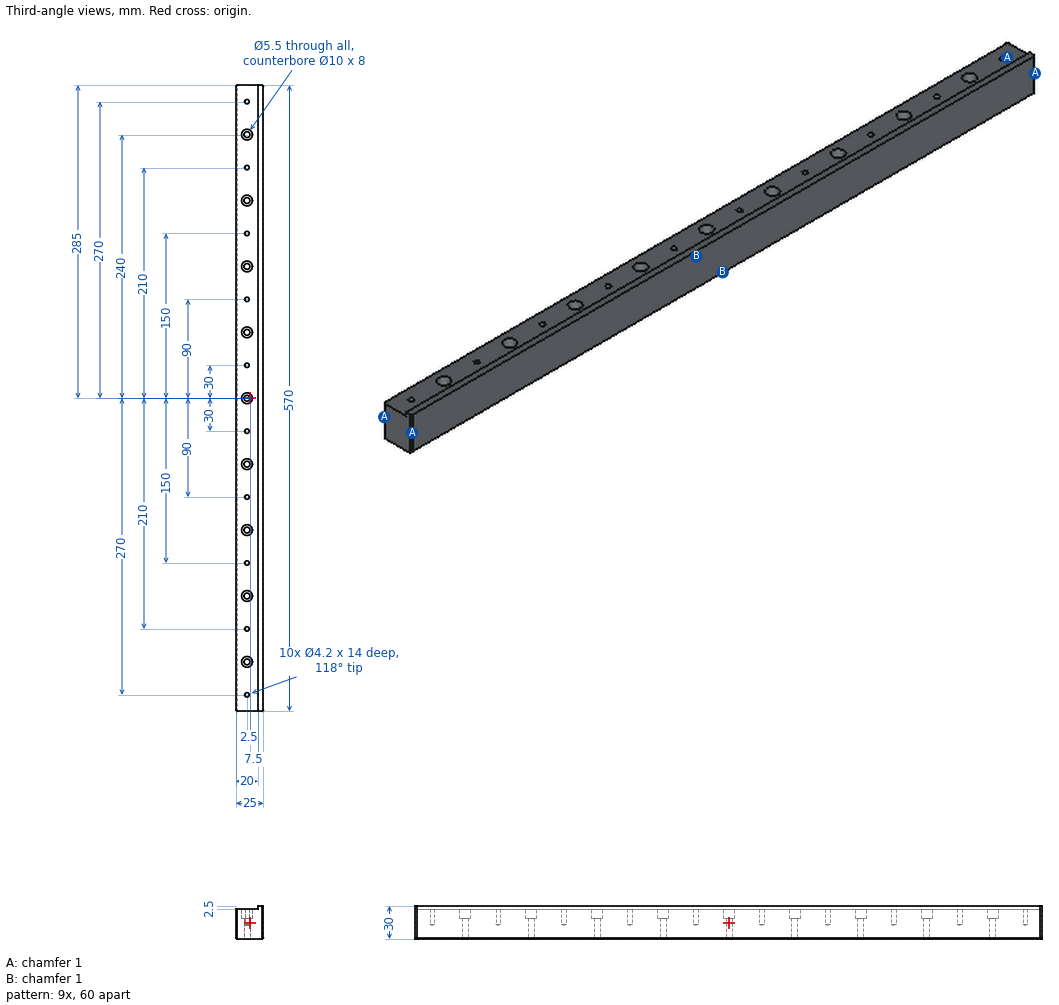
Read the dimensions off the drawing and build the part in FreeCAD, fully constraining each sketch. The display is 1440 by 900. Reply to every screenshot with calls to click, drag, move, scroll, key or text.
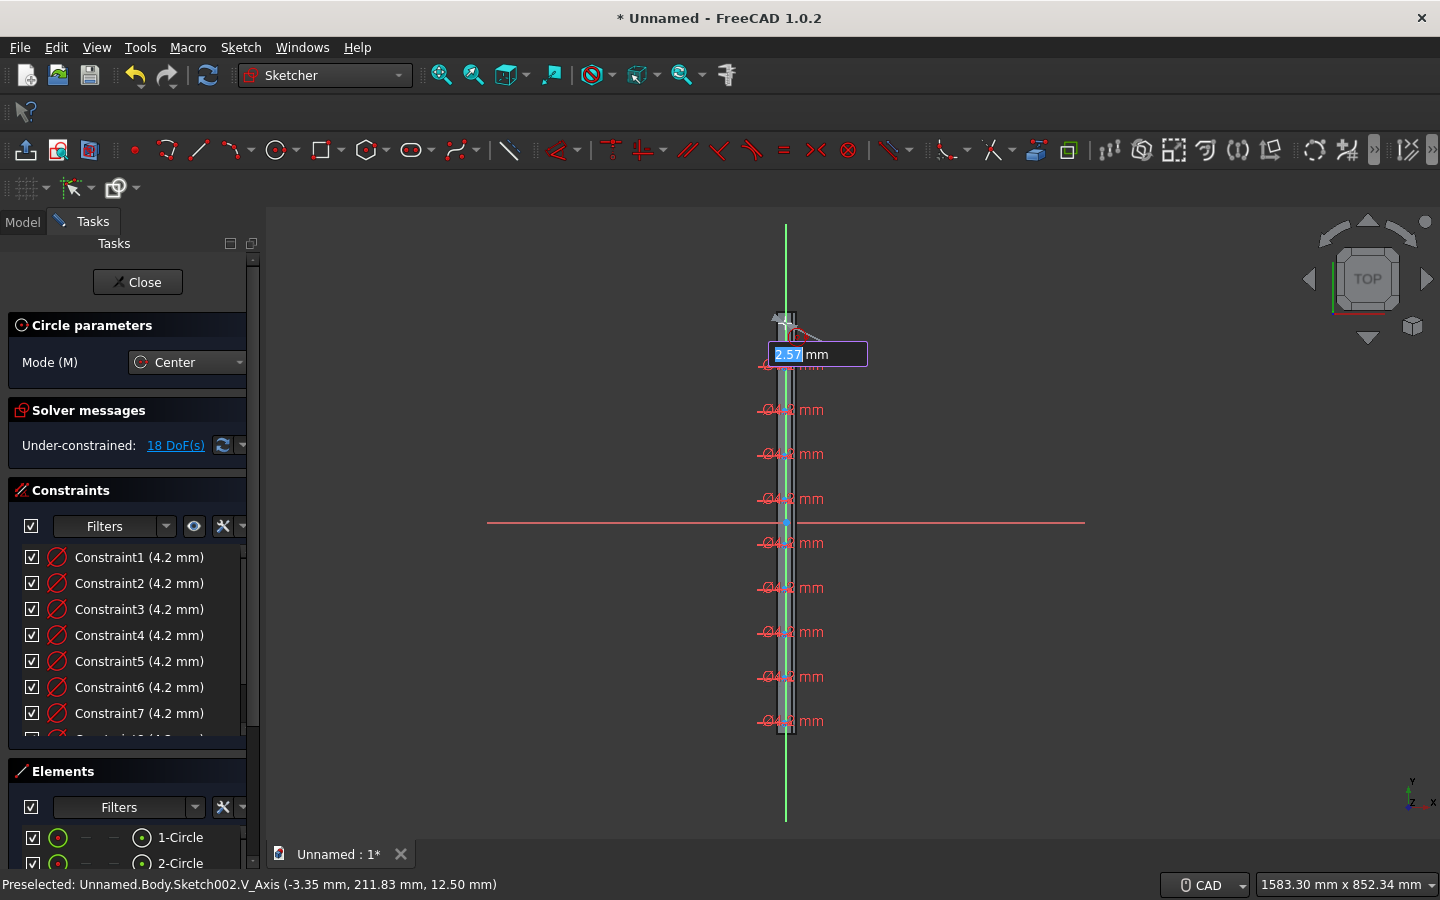
scroll(783, 322, up, 9)
move(783, 319)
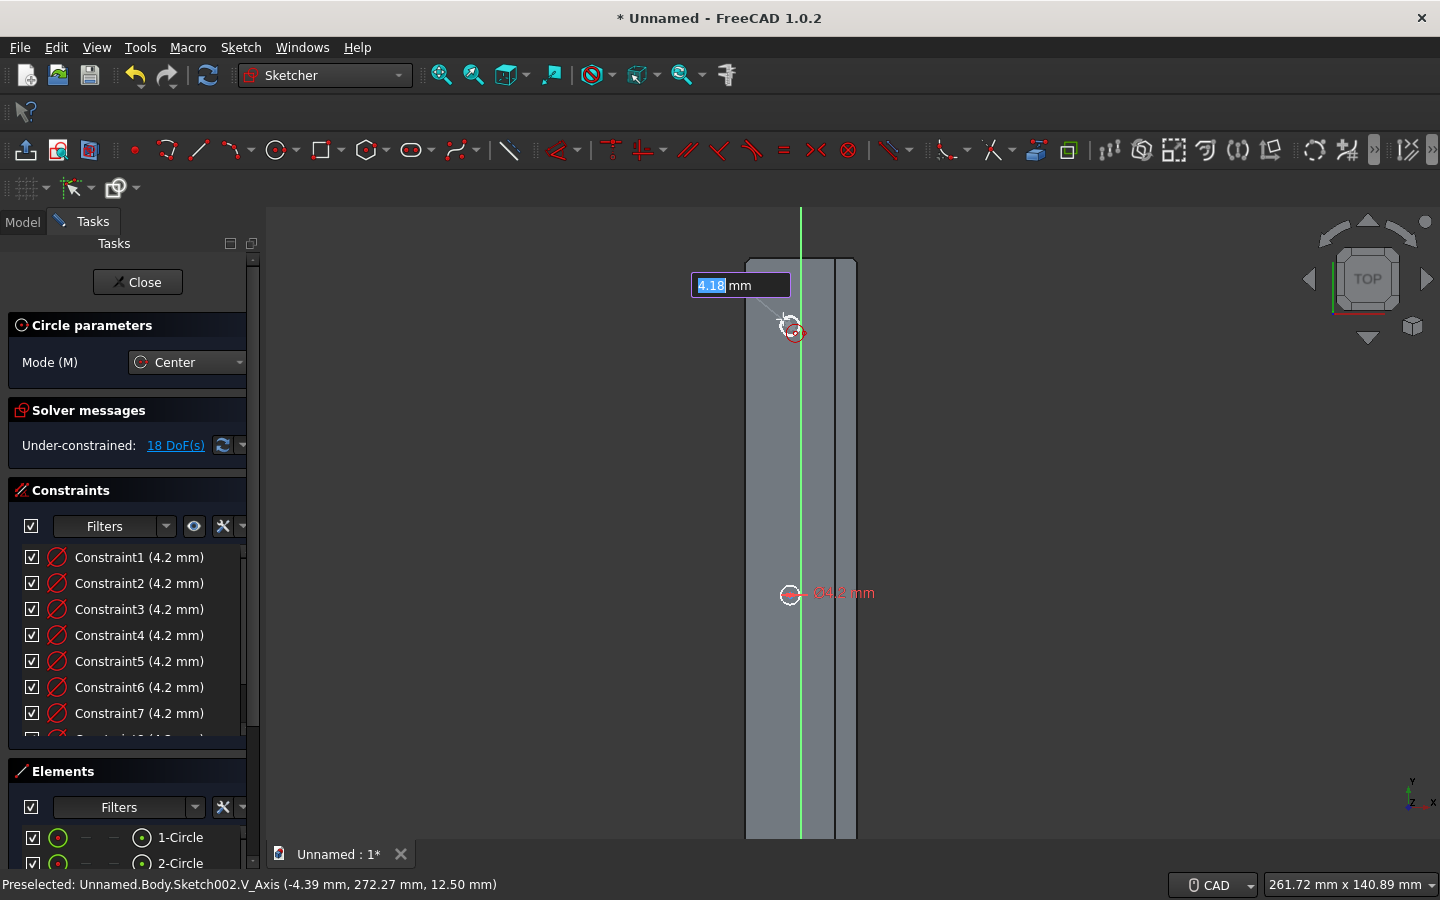
text(4.2)
key(Return)
key(Escape)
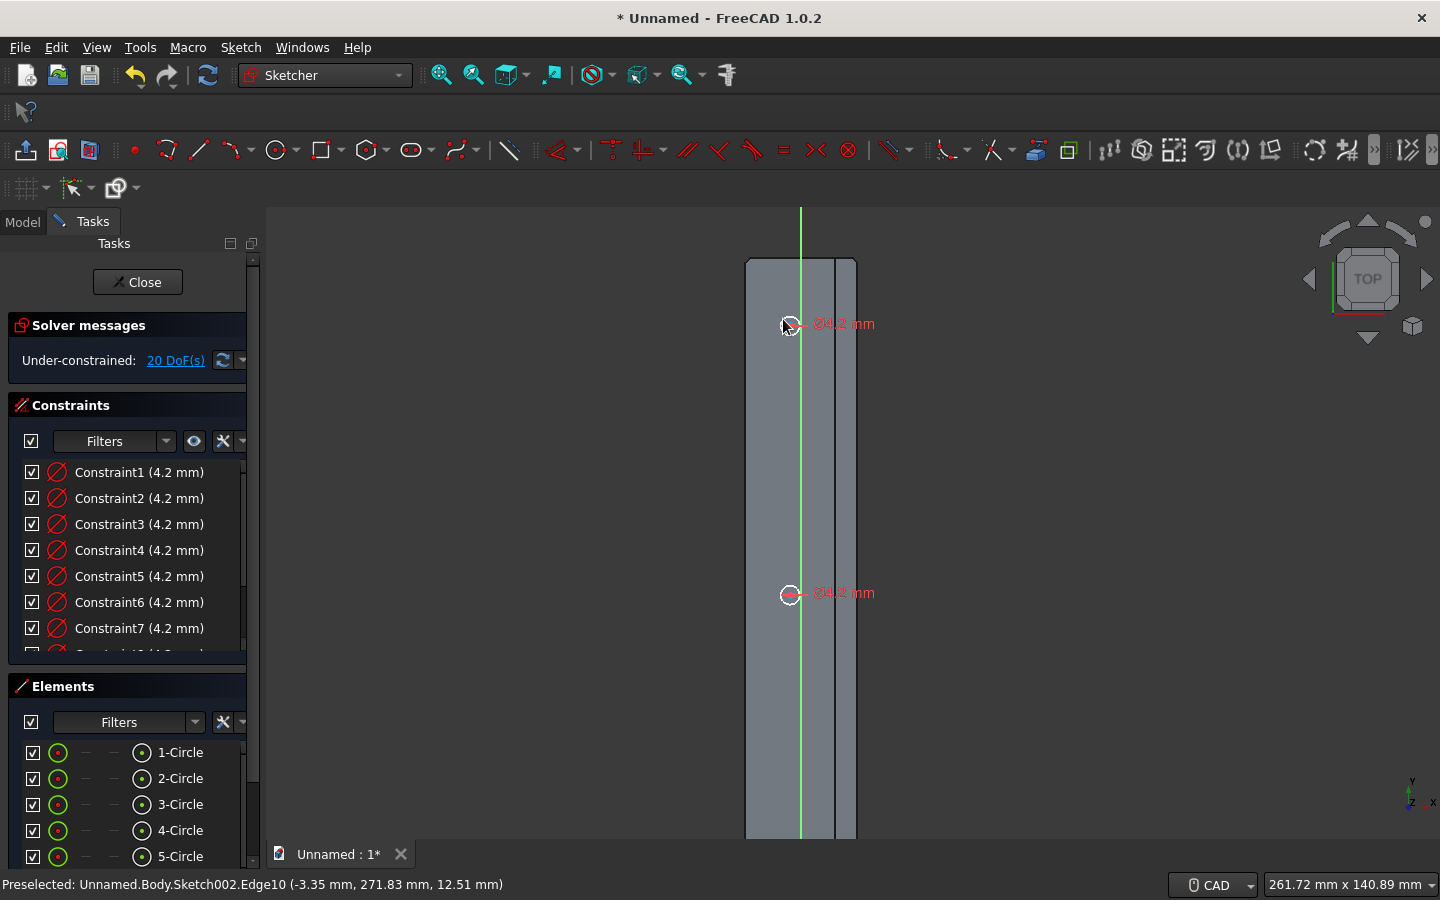
scroll(783, 322, down, 9)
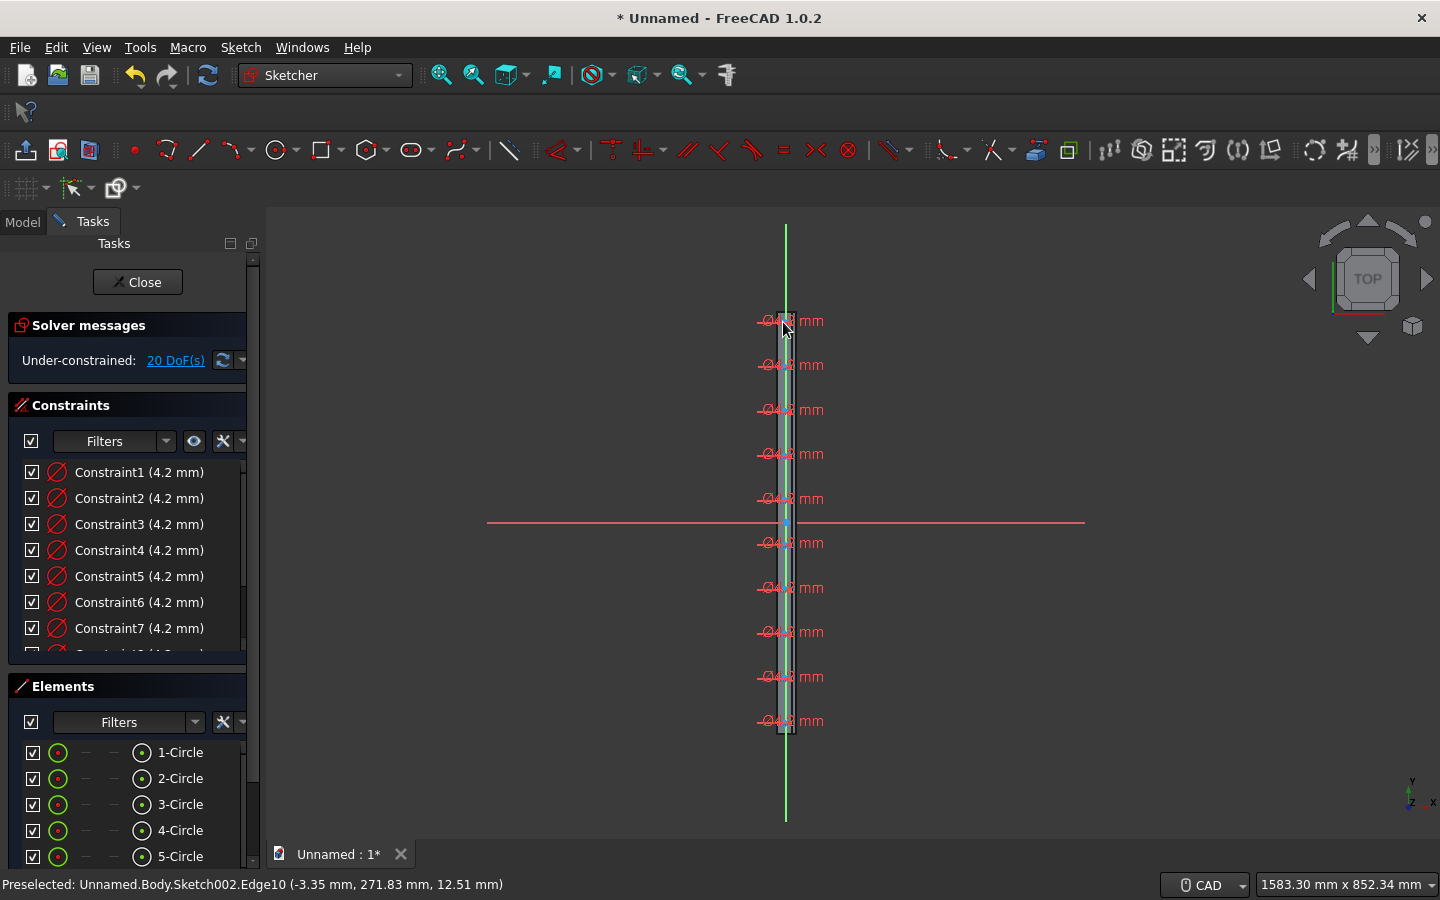
click(785, 723)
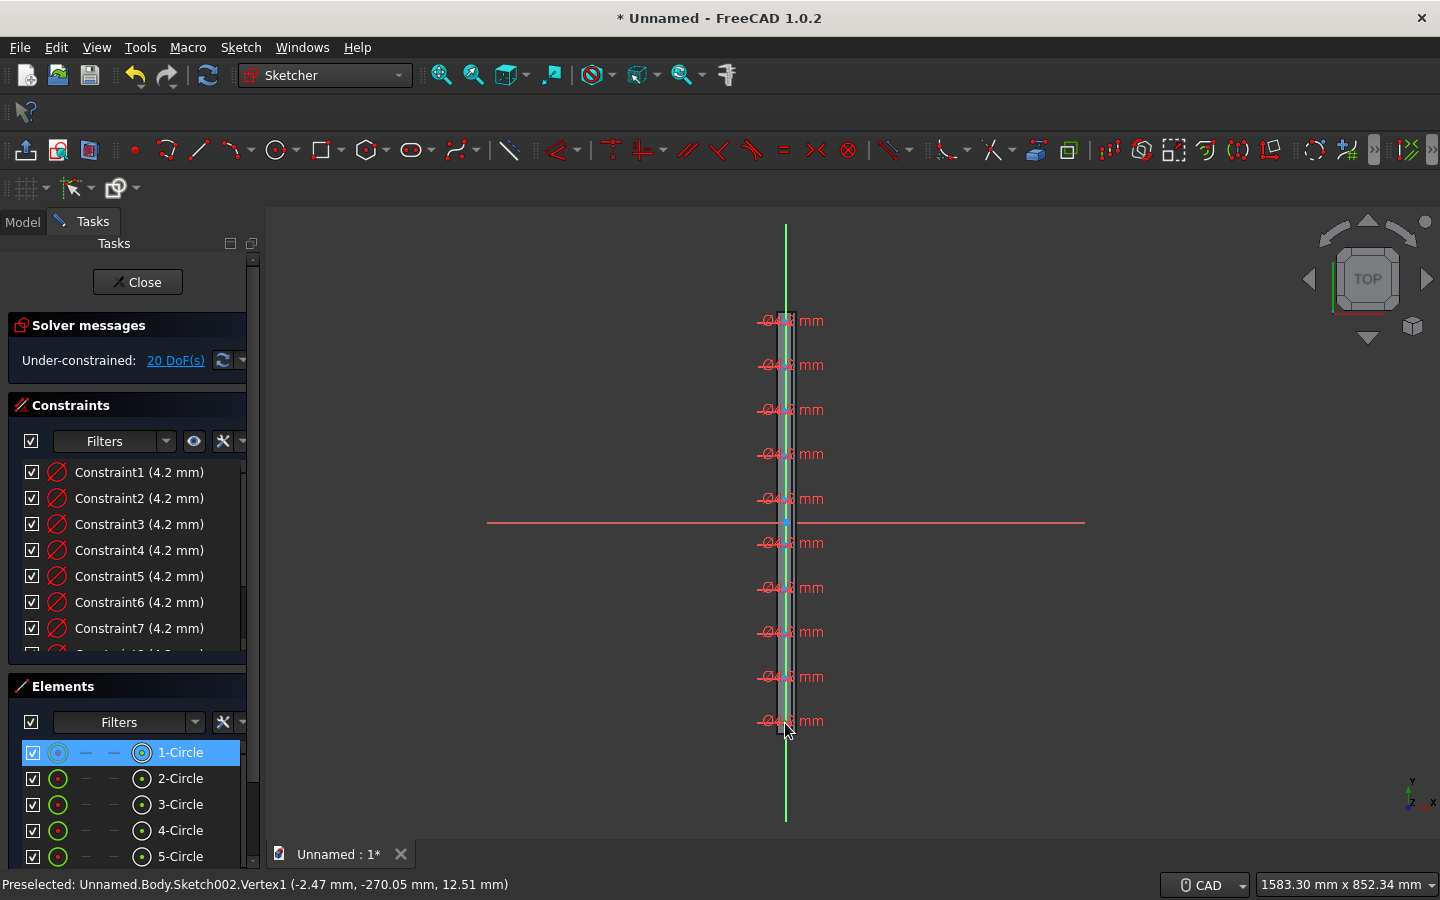
click(785, 679)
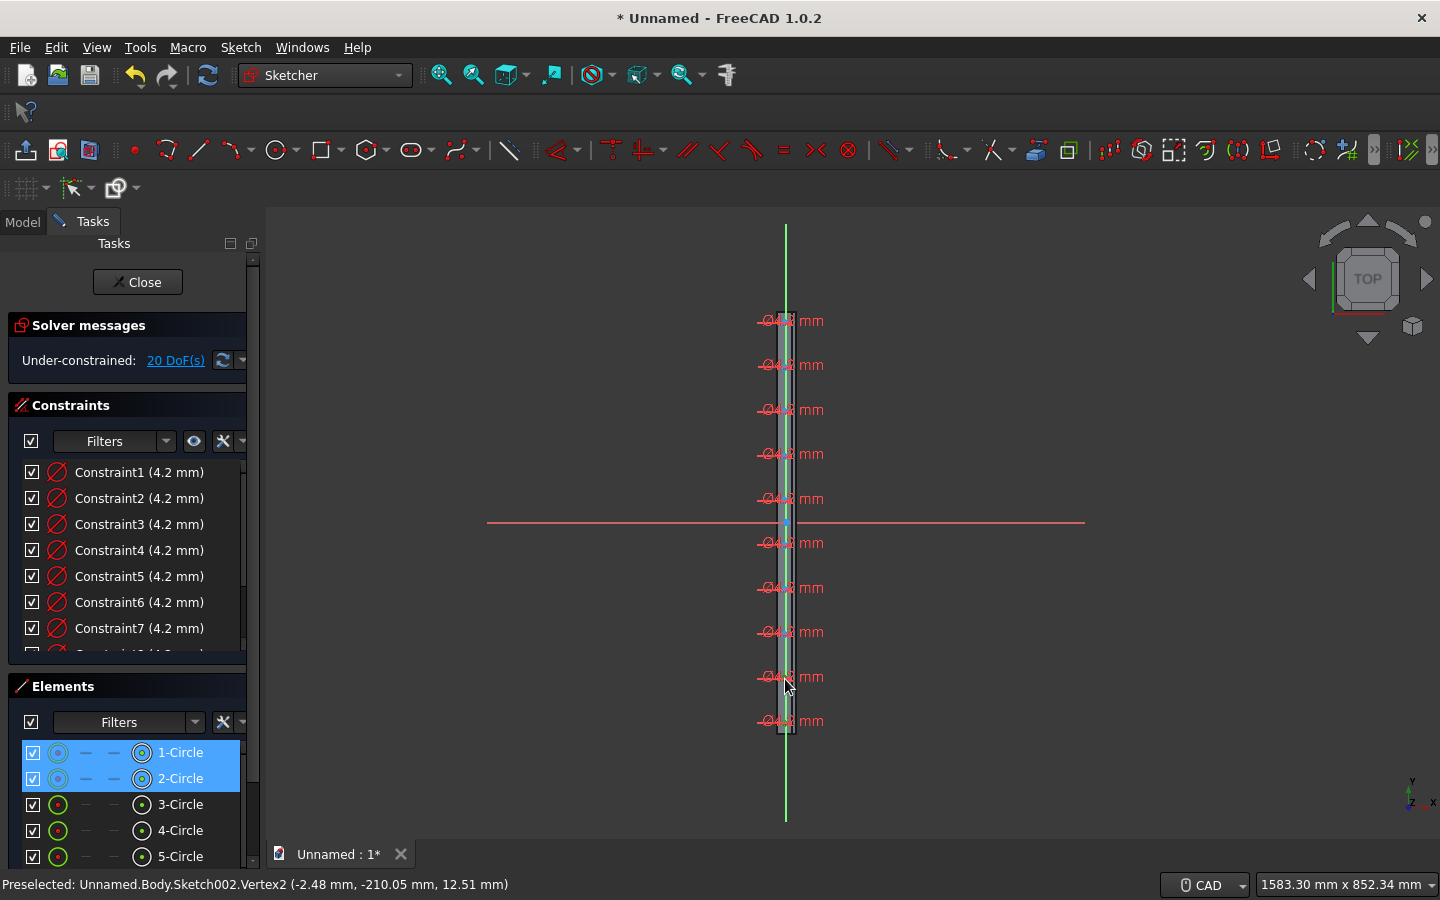
key(v)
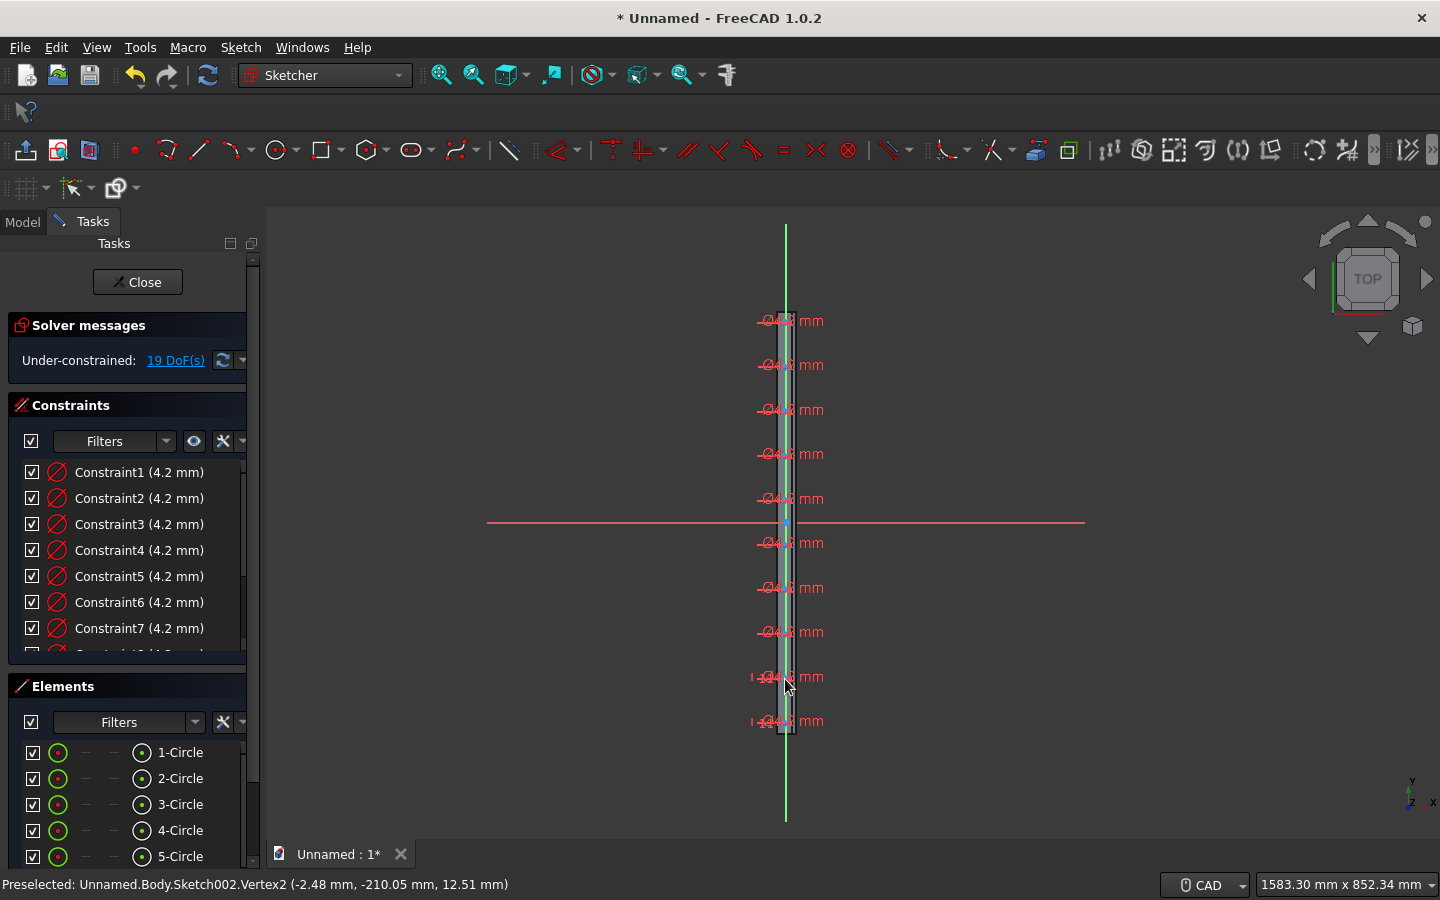
click(785, 679)